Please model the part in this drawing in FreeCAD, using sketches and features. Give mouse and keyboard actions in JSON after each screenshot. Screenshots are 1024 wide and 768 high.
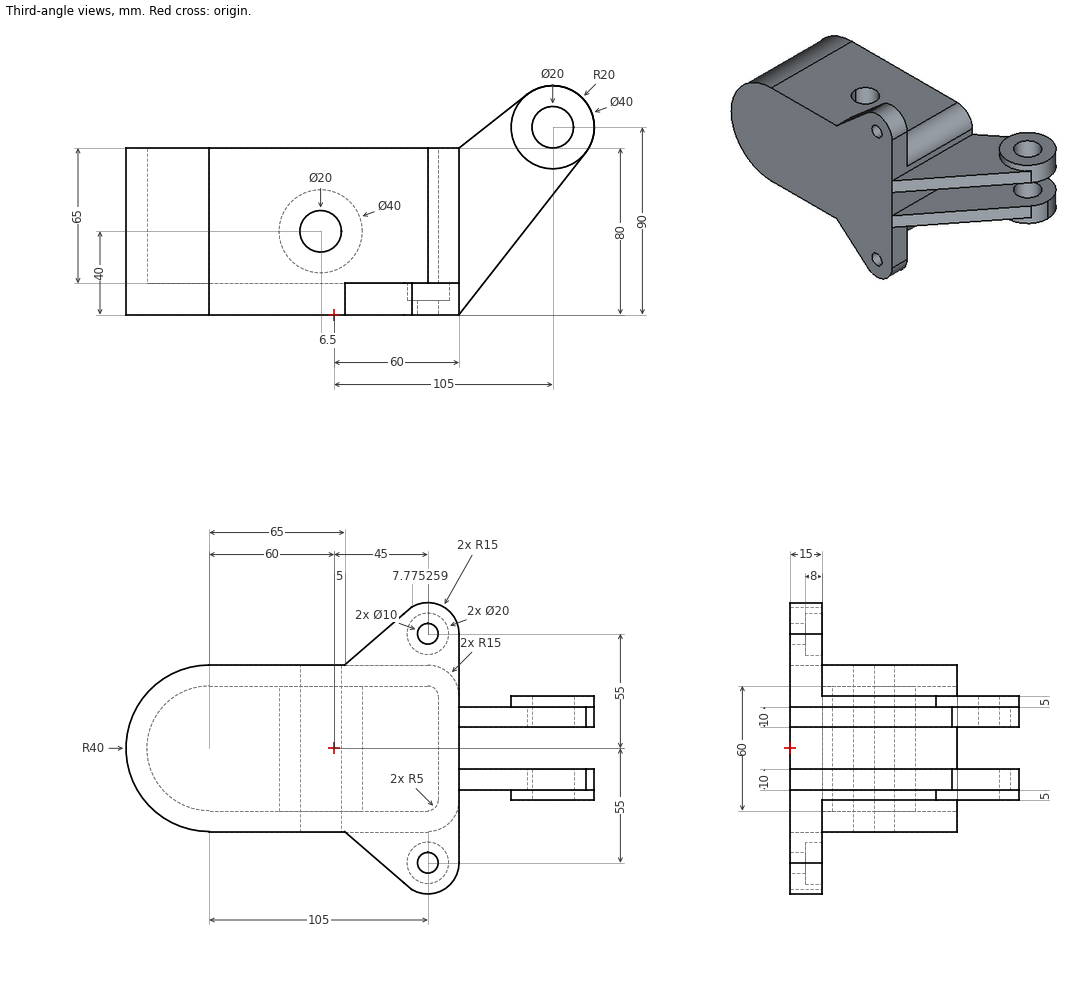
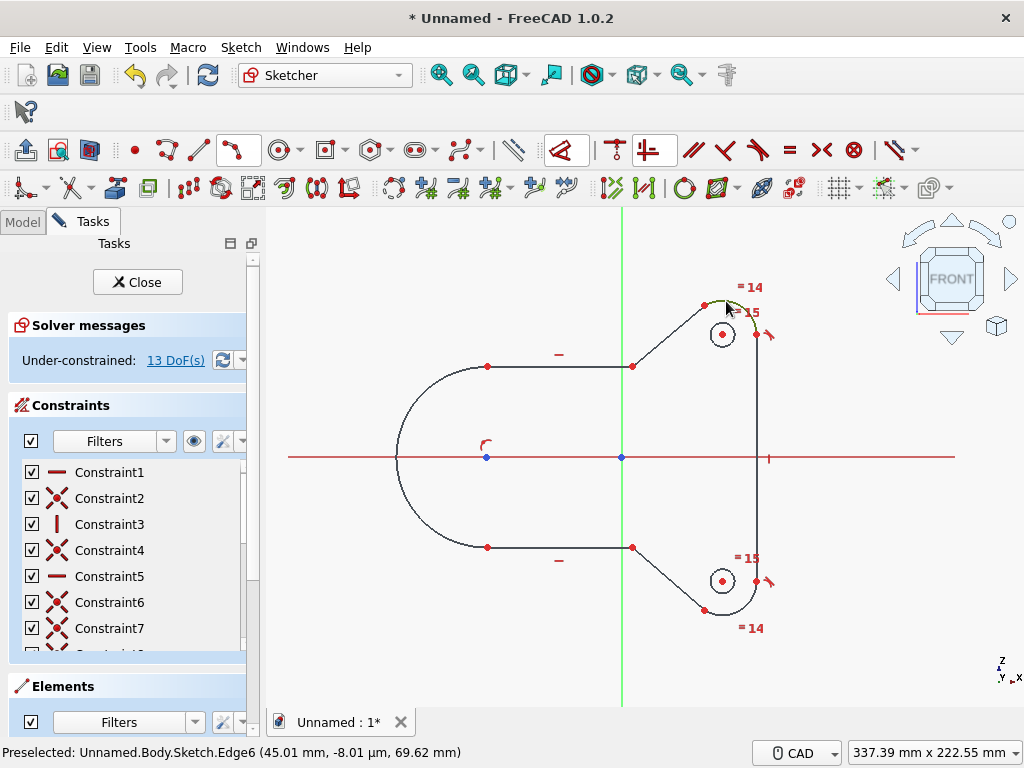
{"action": "key", "text": "k r"}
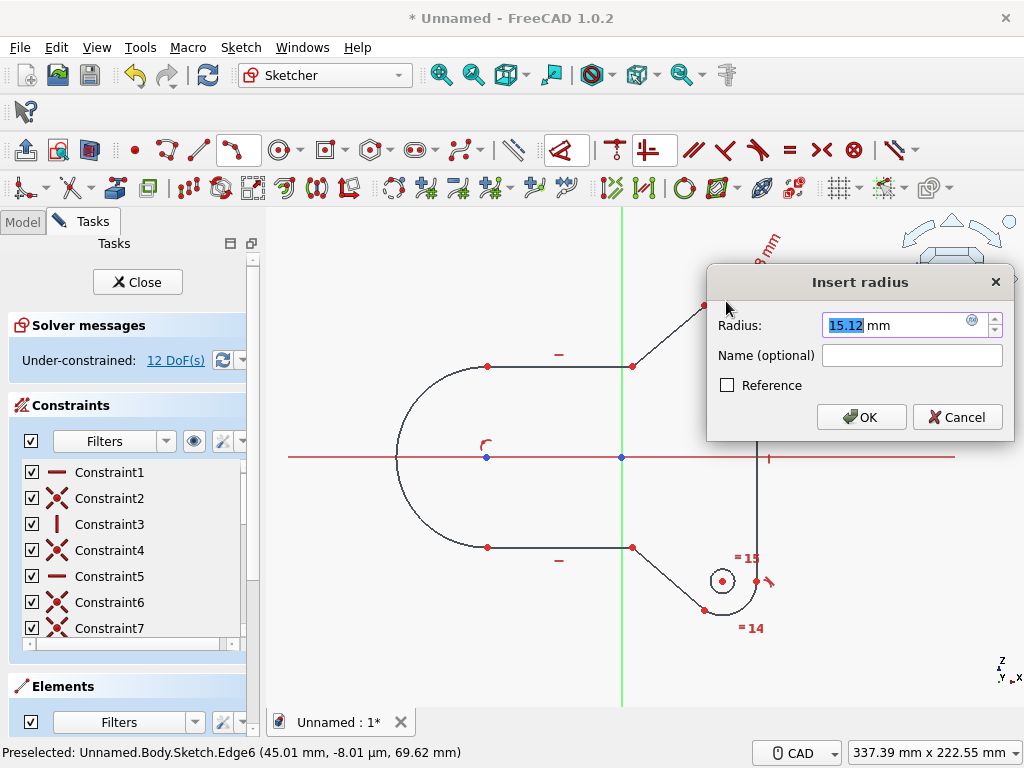
{"action": "type", "text": "15"}
{"action": "key", "text": "Return"}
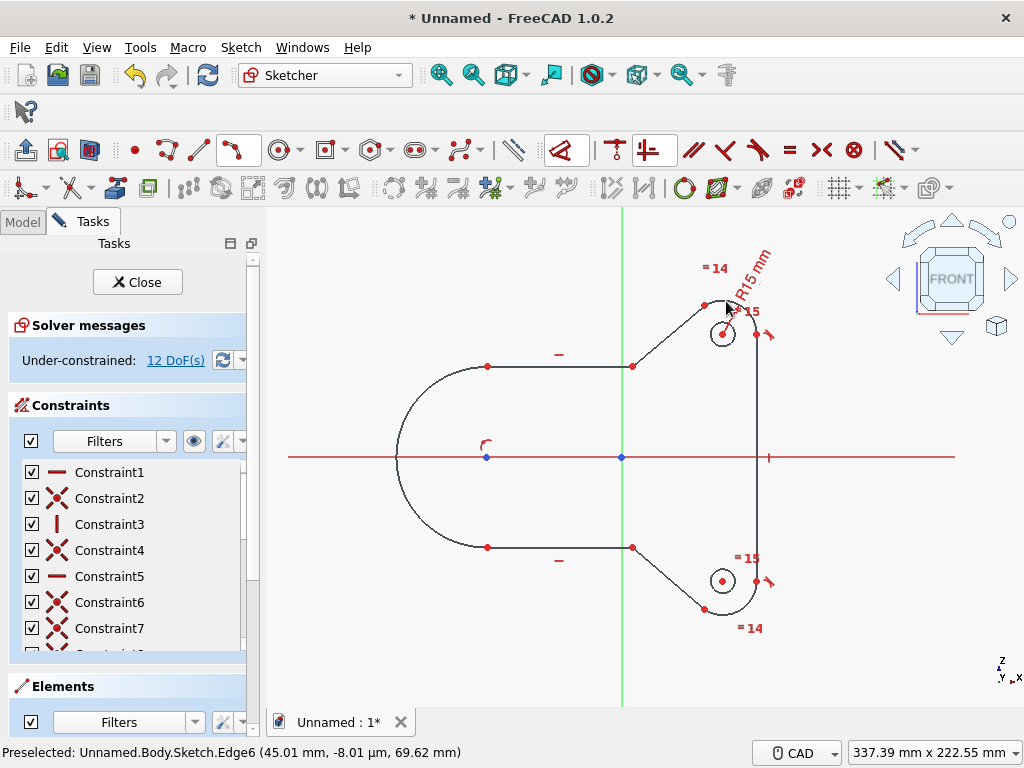
{"action": "left_click", "coordinate": [414, 404]}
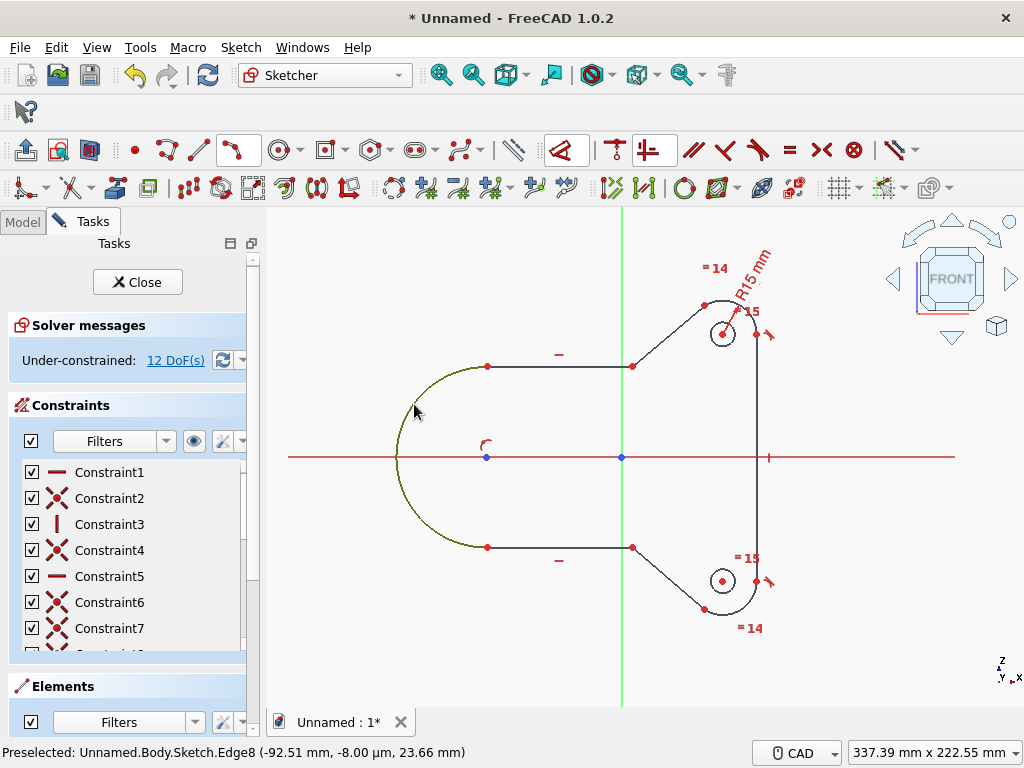
{"action": "left_click", "coordinate": [584, 150]}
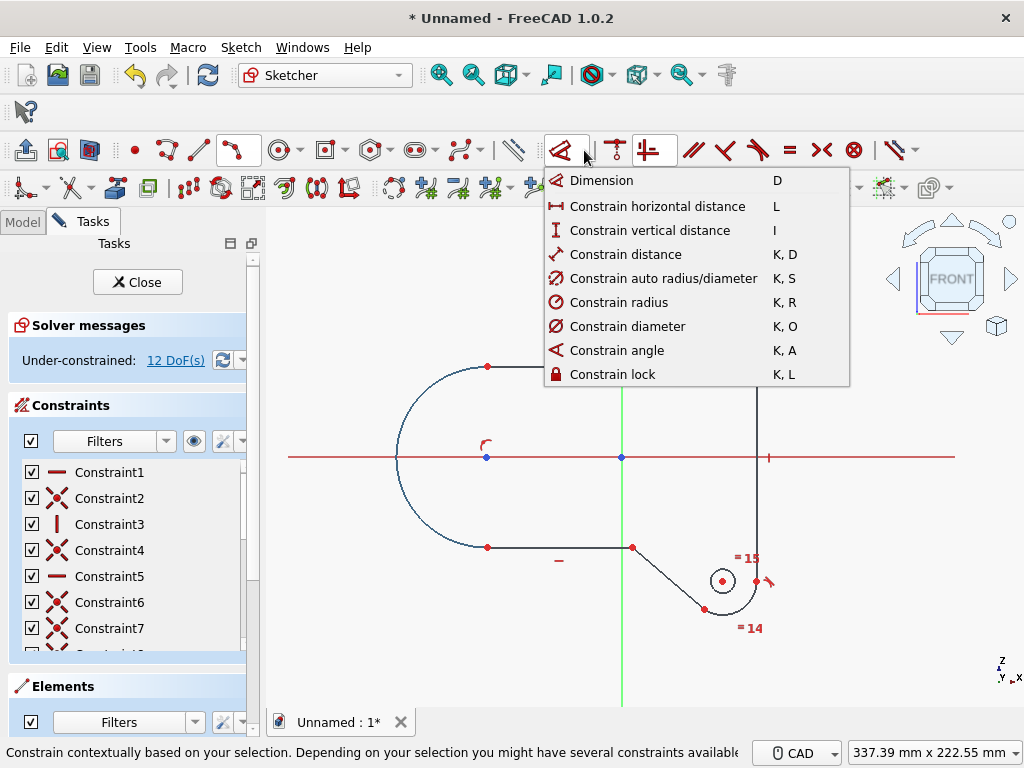
{"action": "left_click", "coordinate": [697, 302]}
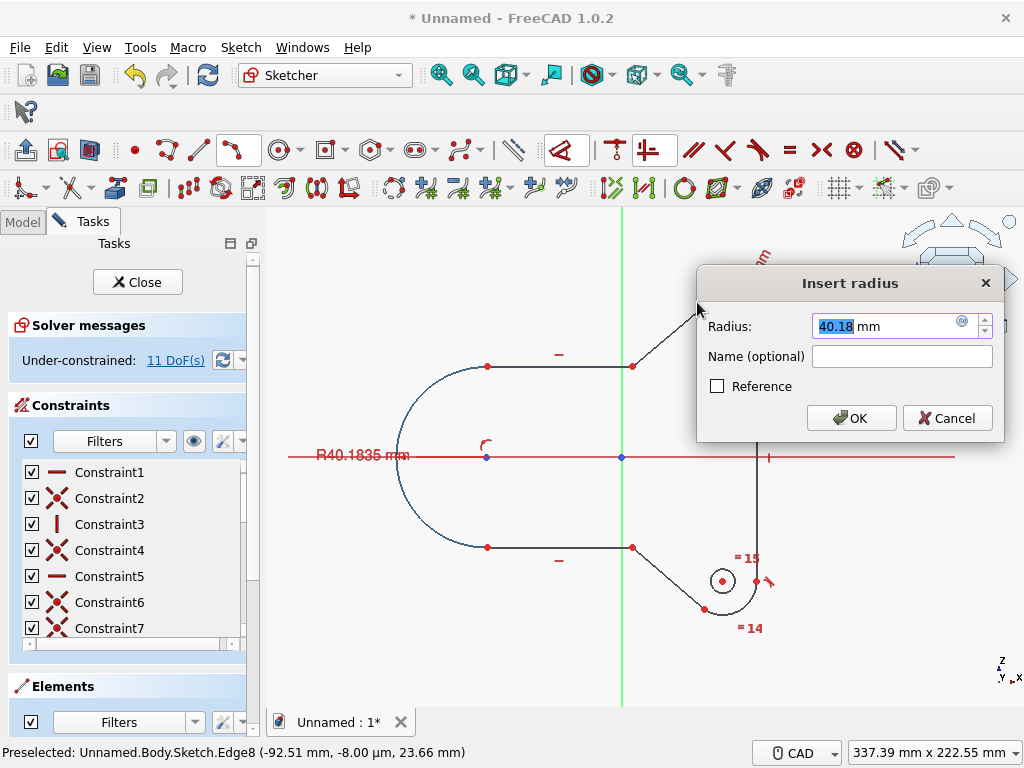
{"action": "type", "text": "40"}
{"action": "key", "text": "Return"}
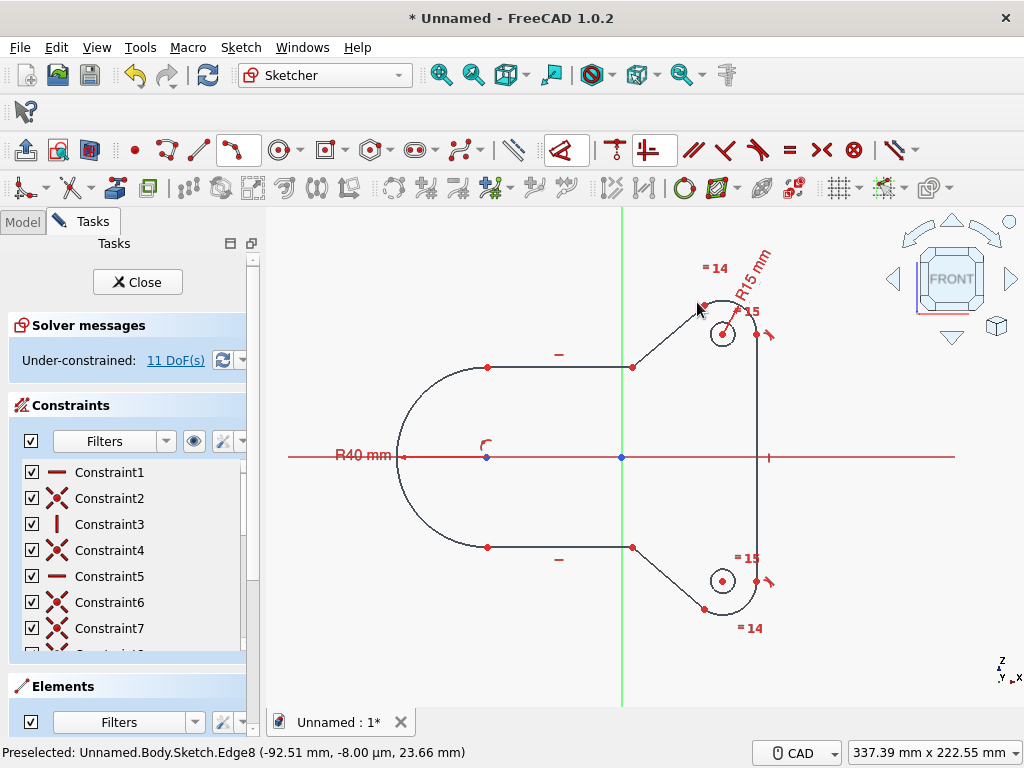
{"action": "scroll", "coordinate": [731, 326], "scroll_direction": "up", "scroll_amount": 3}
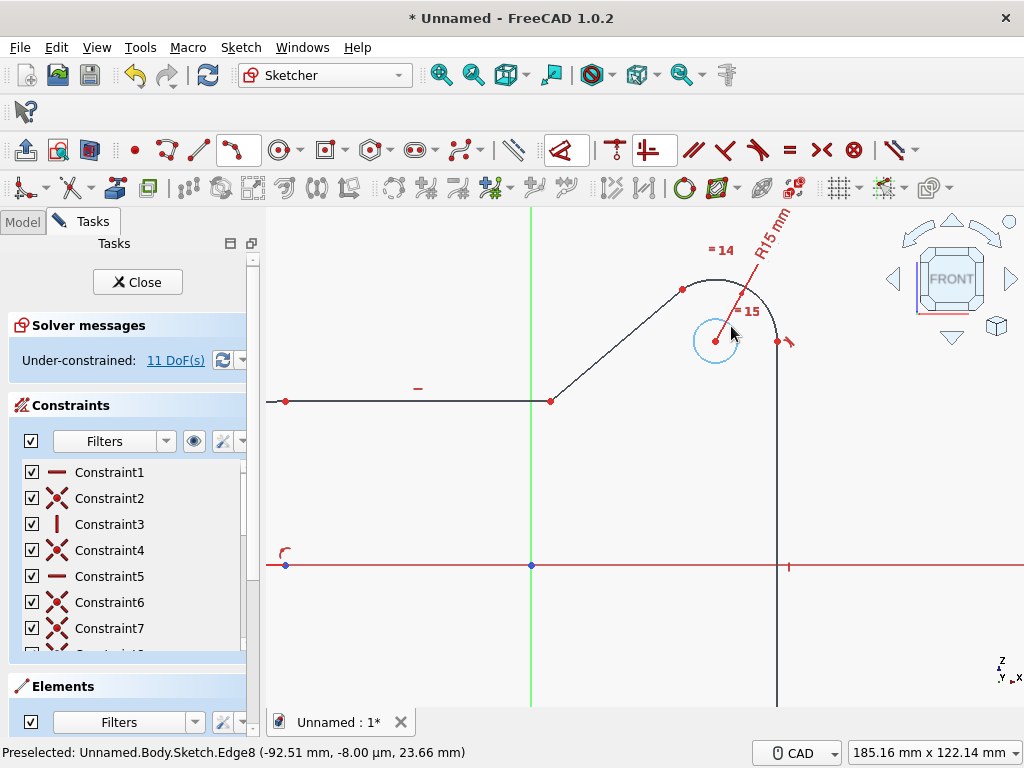
{"action": "left_click", "coordinate": [731, 326]}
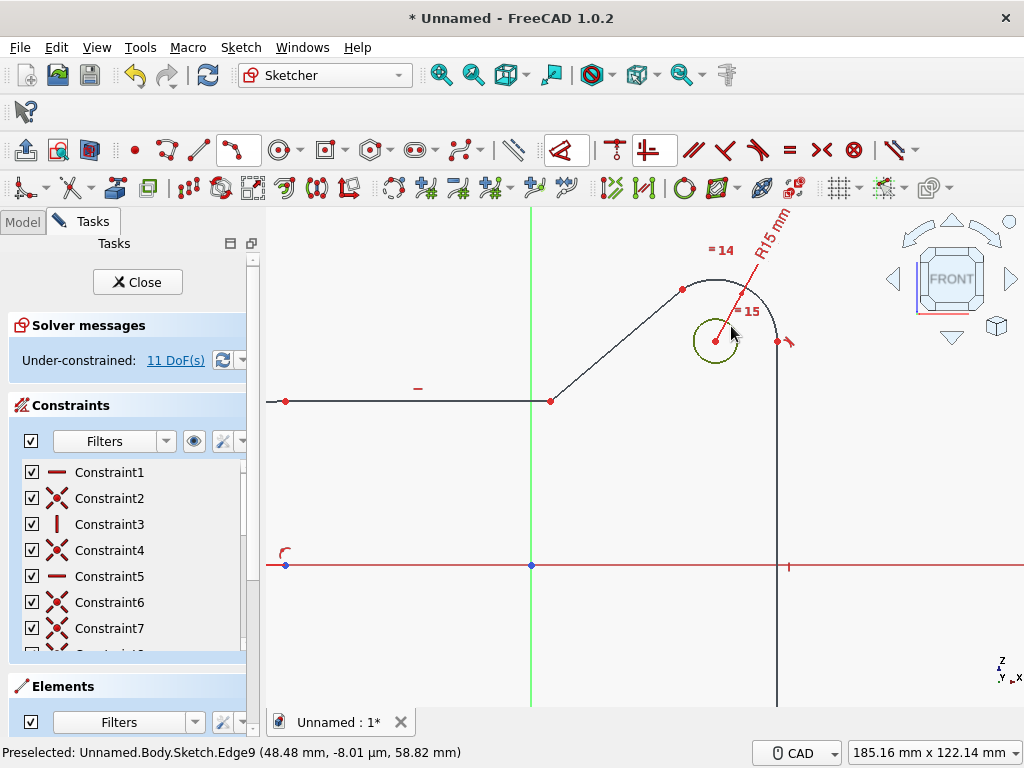
{"action": "key", "text": "k o"}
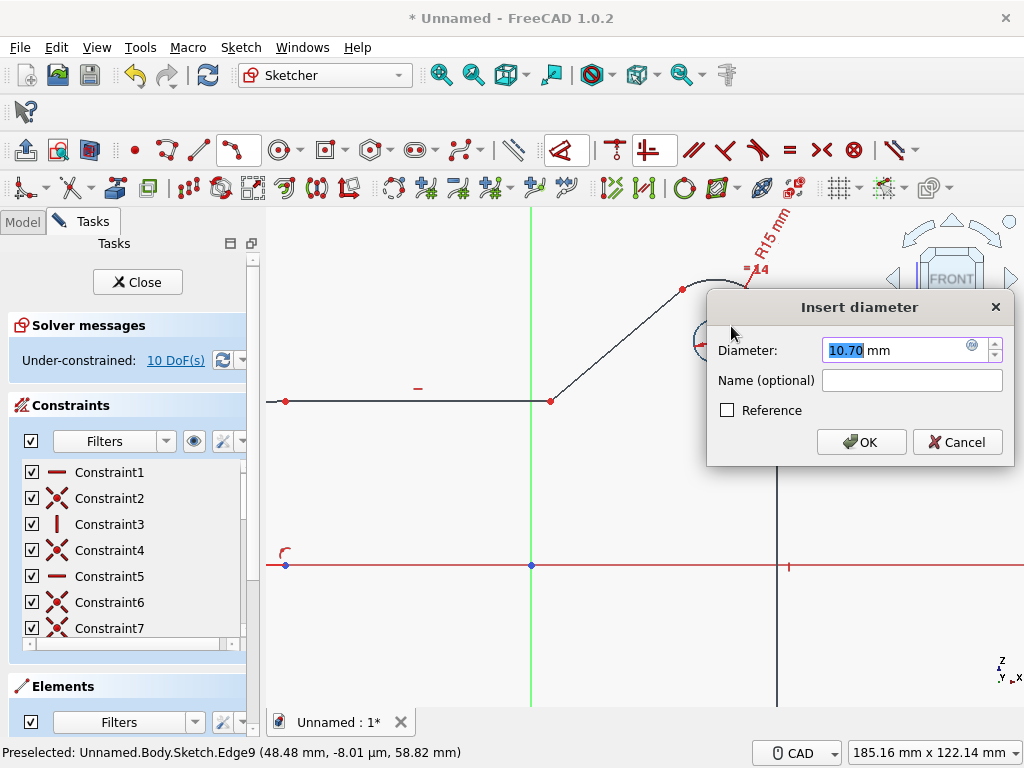
{"action": "type", "text": "10"}
{"action": "key", "text": "Return"}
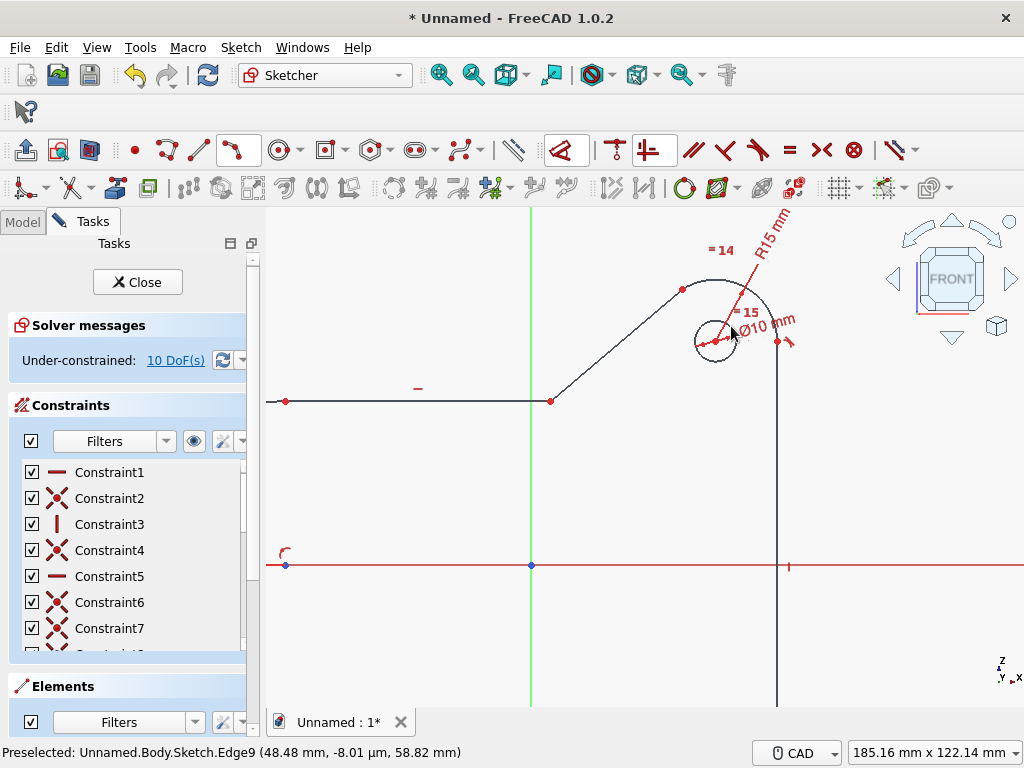
{"action": "left_click", "coordinate": [365, 401]}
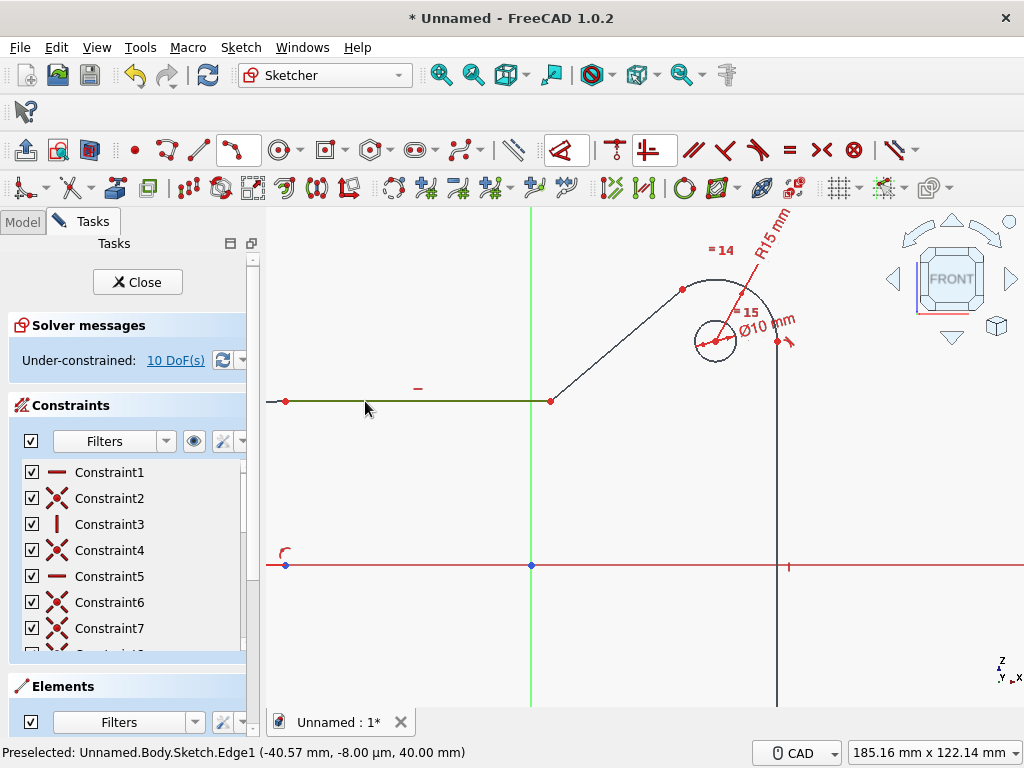
{"action": "left_click", "coordinate": [584, 150]}